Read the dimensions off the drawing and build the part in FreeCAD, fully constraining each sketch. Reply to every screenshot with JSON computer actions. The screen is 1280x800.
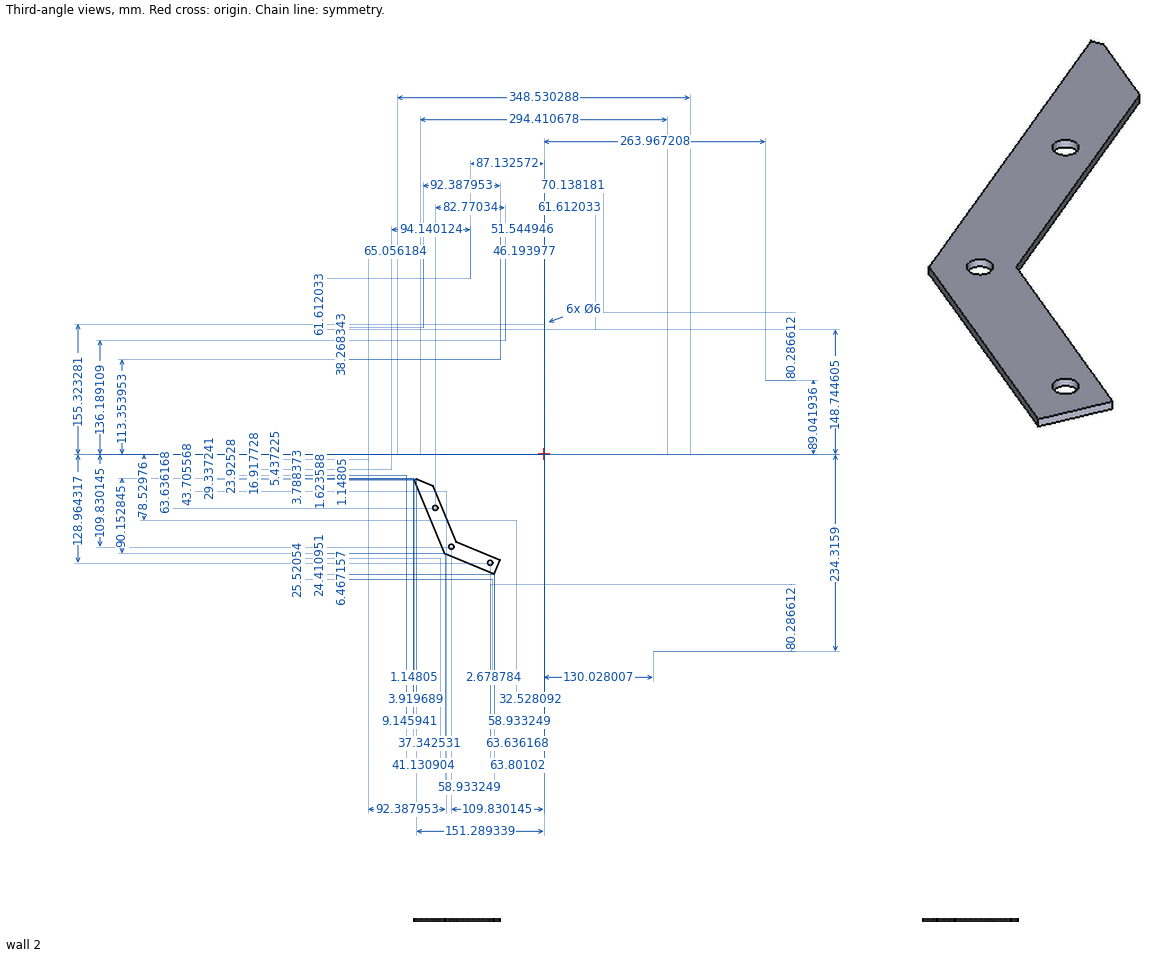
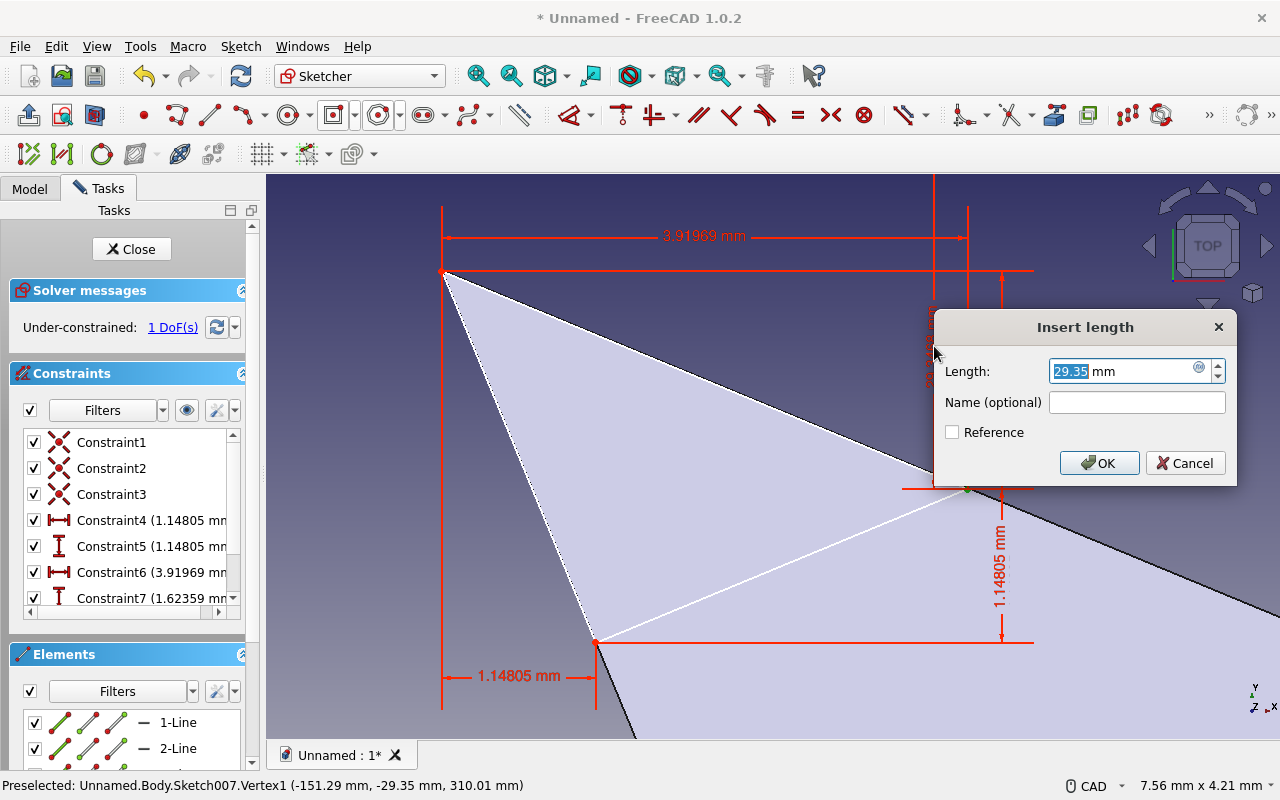
{"action": "type", "text": "29.337241"}
{"action": "key", "text": "Return"}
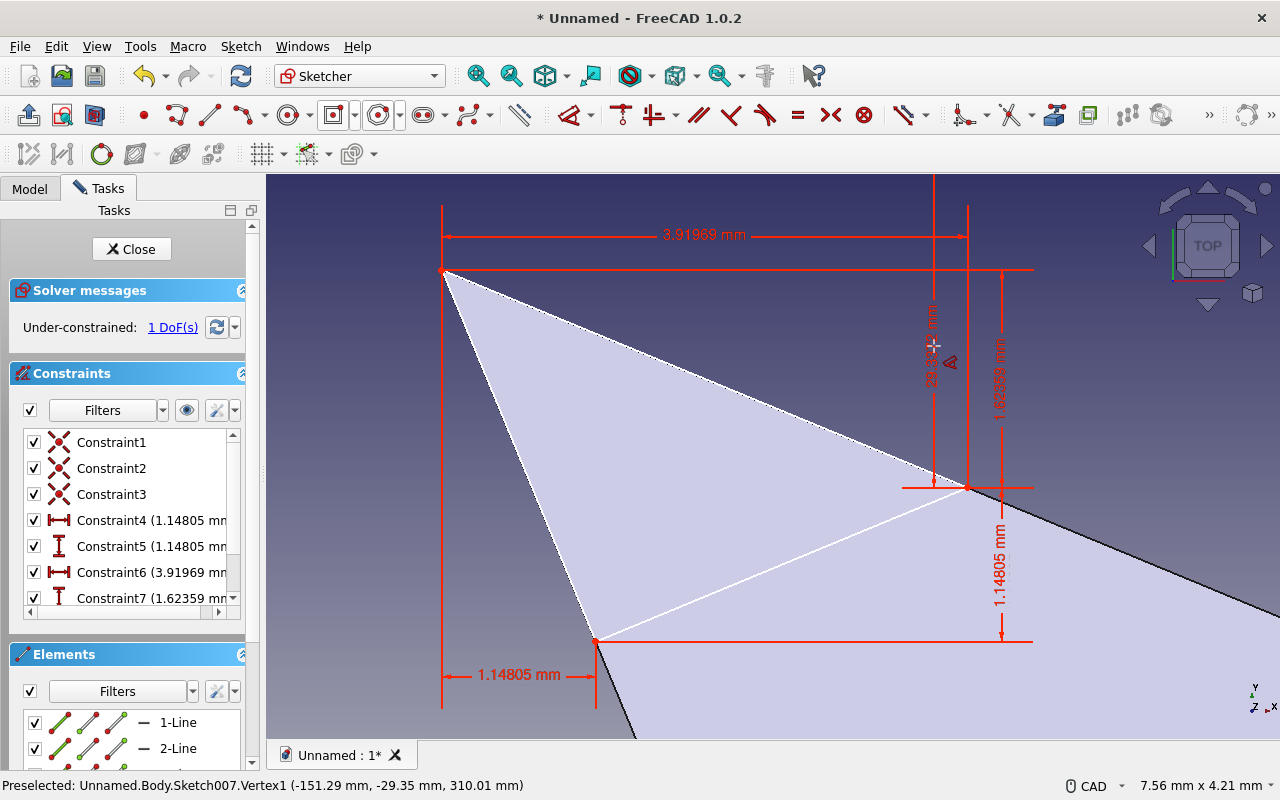
{"action": "left_click", "coordinate": [968, 488]}
{"action": "left_click", "coordinate": [1041, 522]}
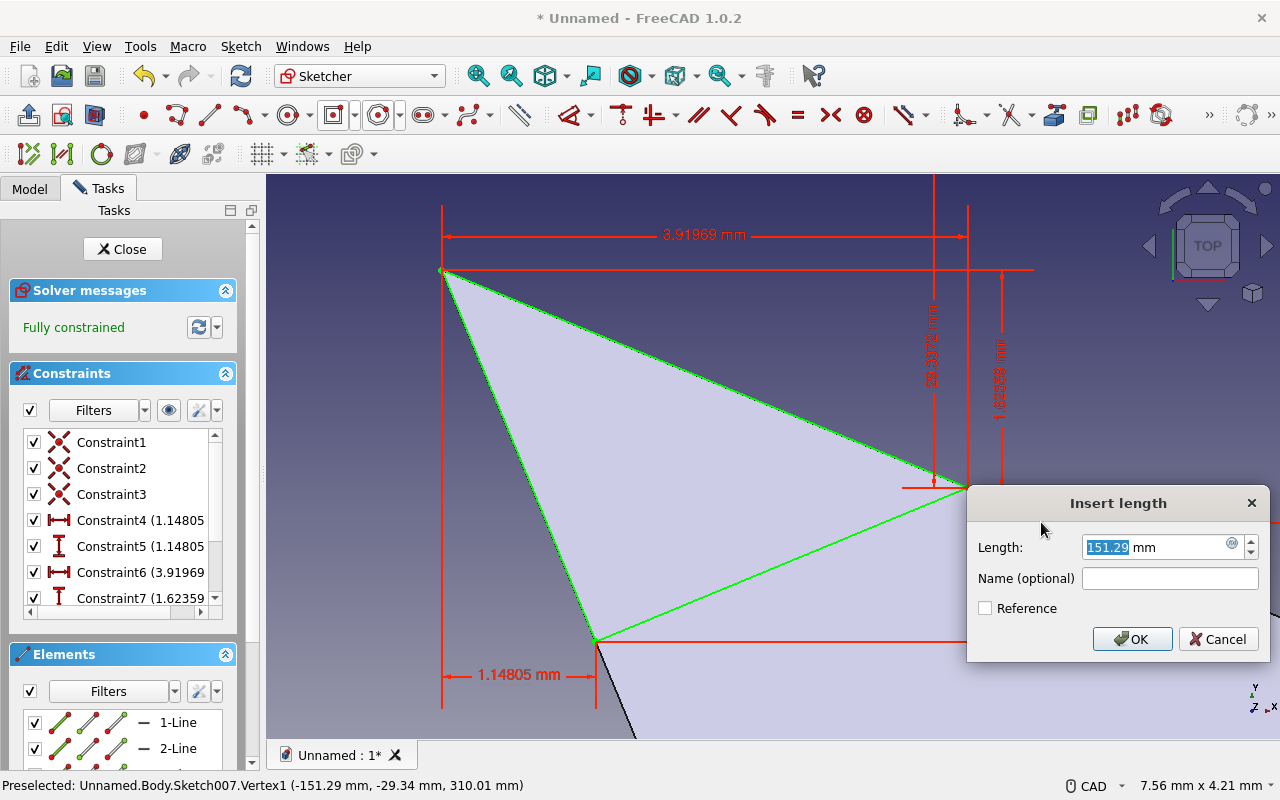
{"action": "type", "text": "151.289339"}
{"action": "key", "text": "Return"}
{"action": "key", "text": "Escape"}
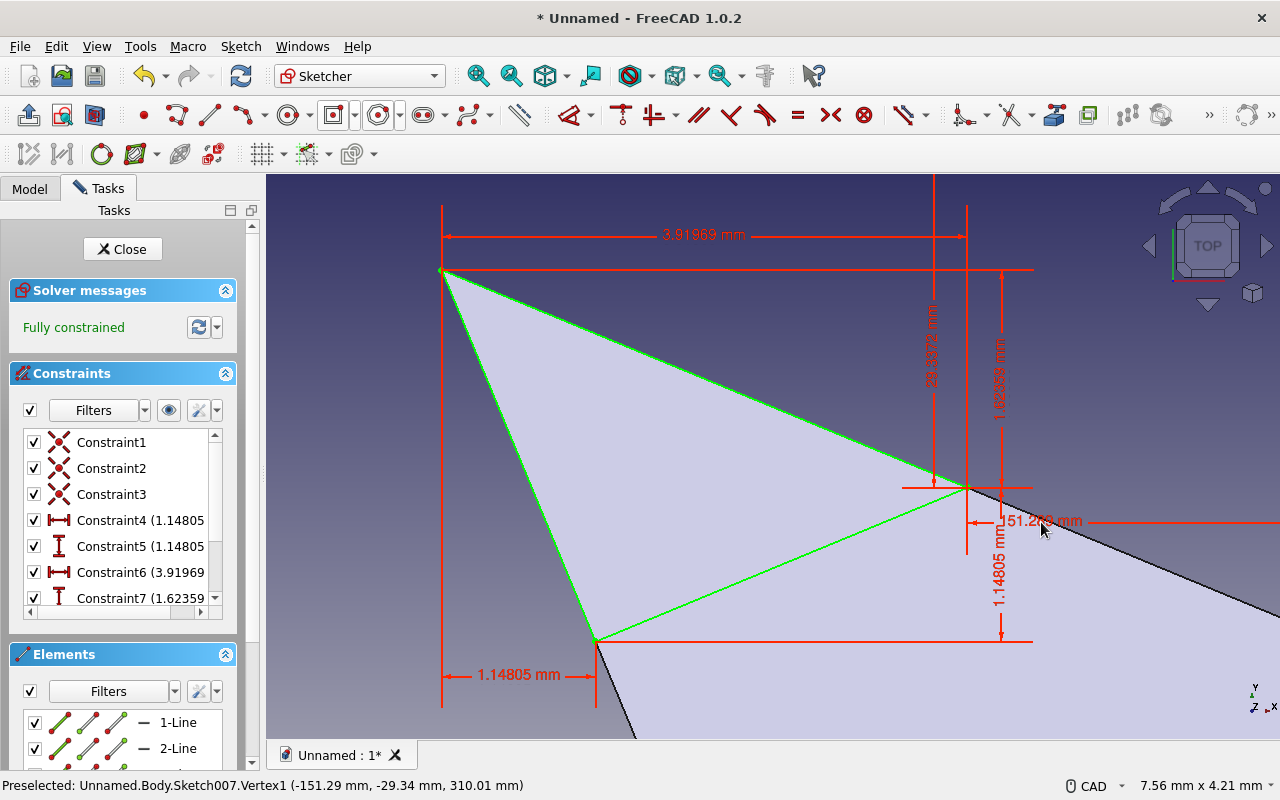
{"action": "left_click", "coordinate": [123, 249]}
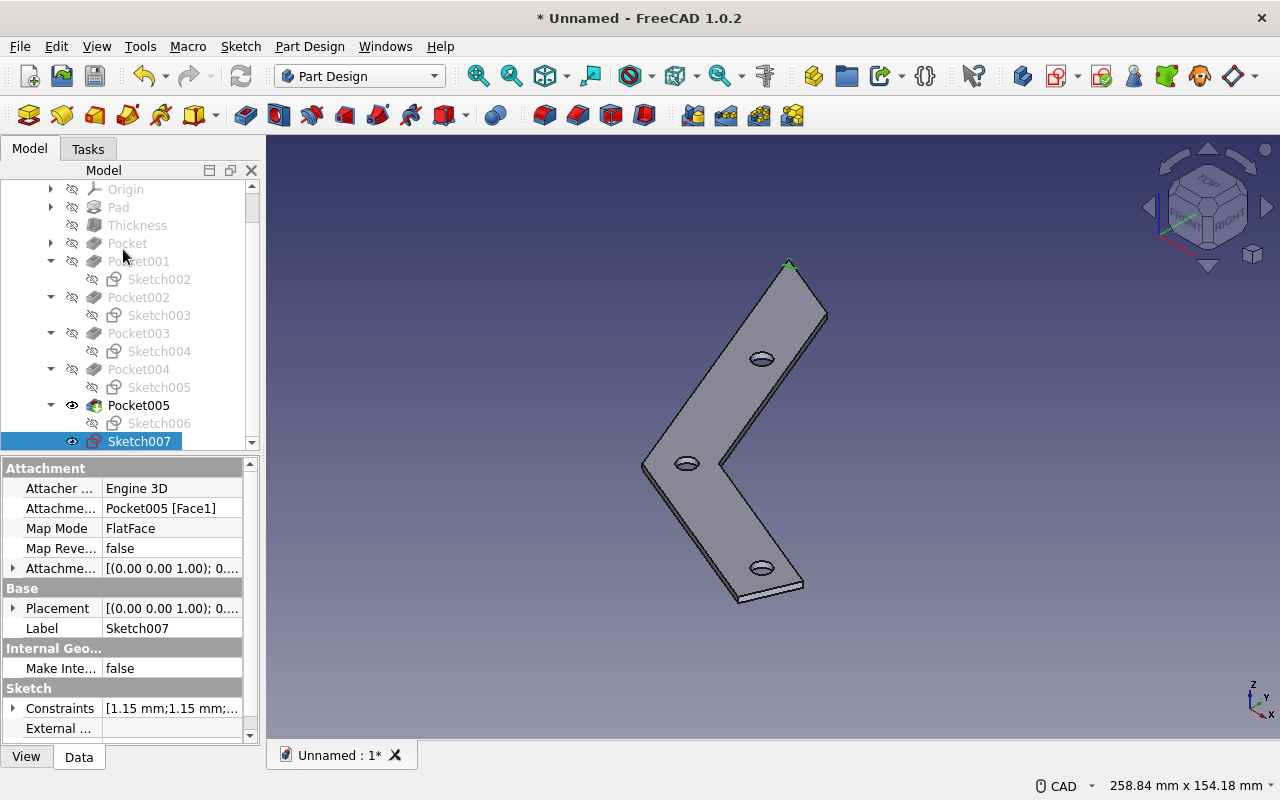
{"action": "left_click", "coordinate": [246, 116]}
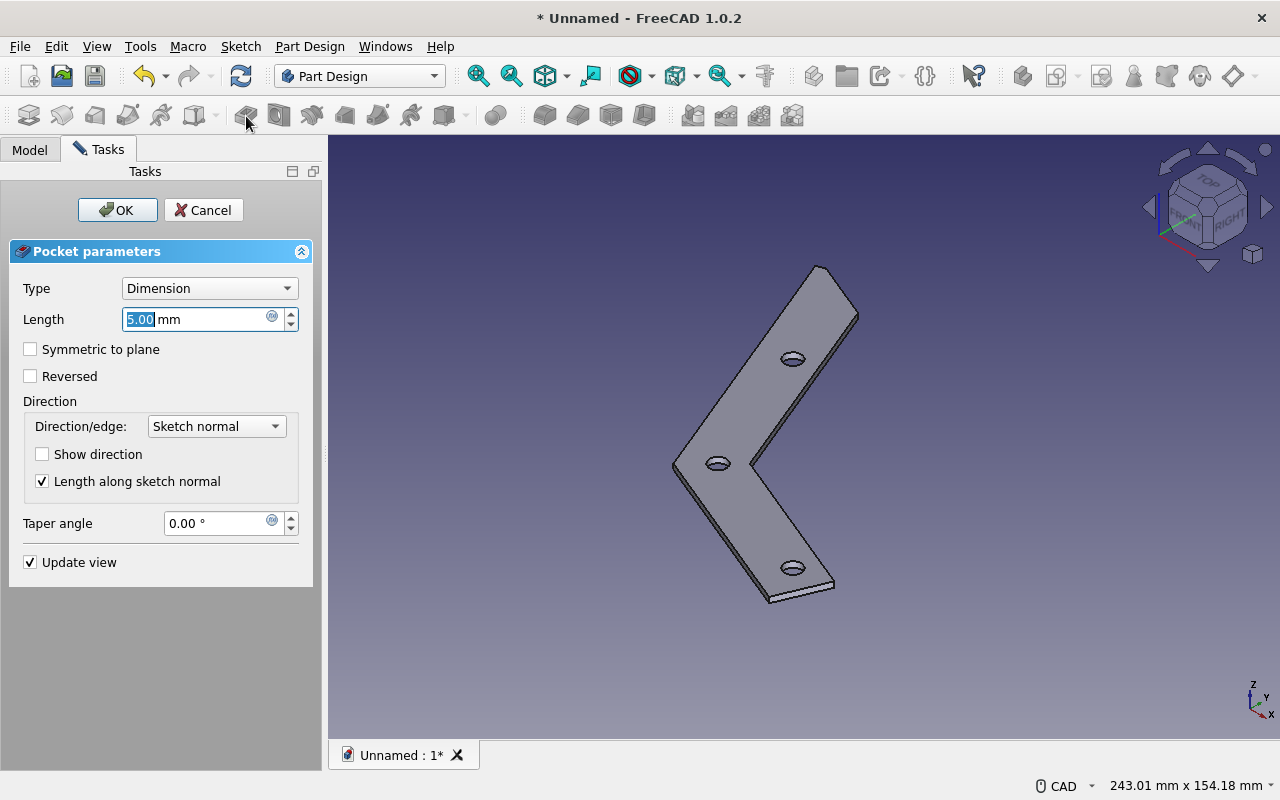
{"action": "left_click", "coordinate": [210, 288]}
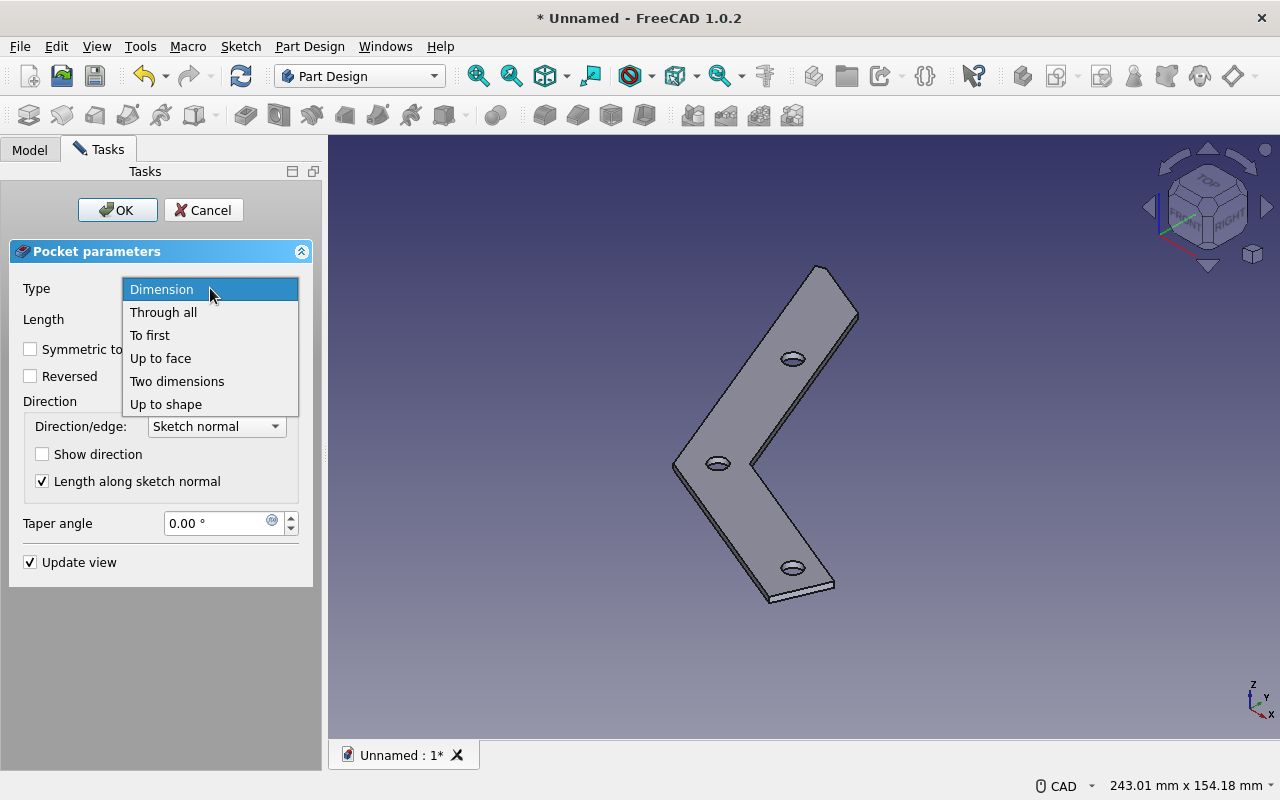
{"action": "left_click", "coordinate": [208, 312]}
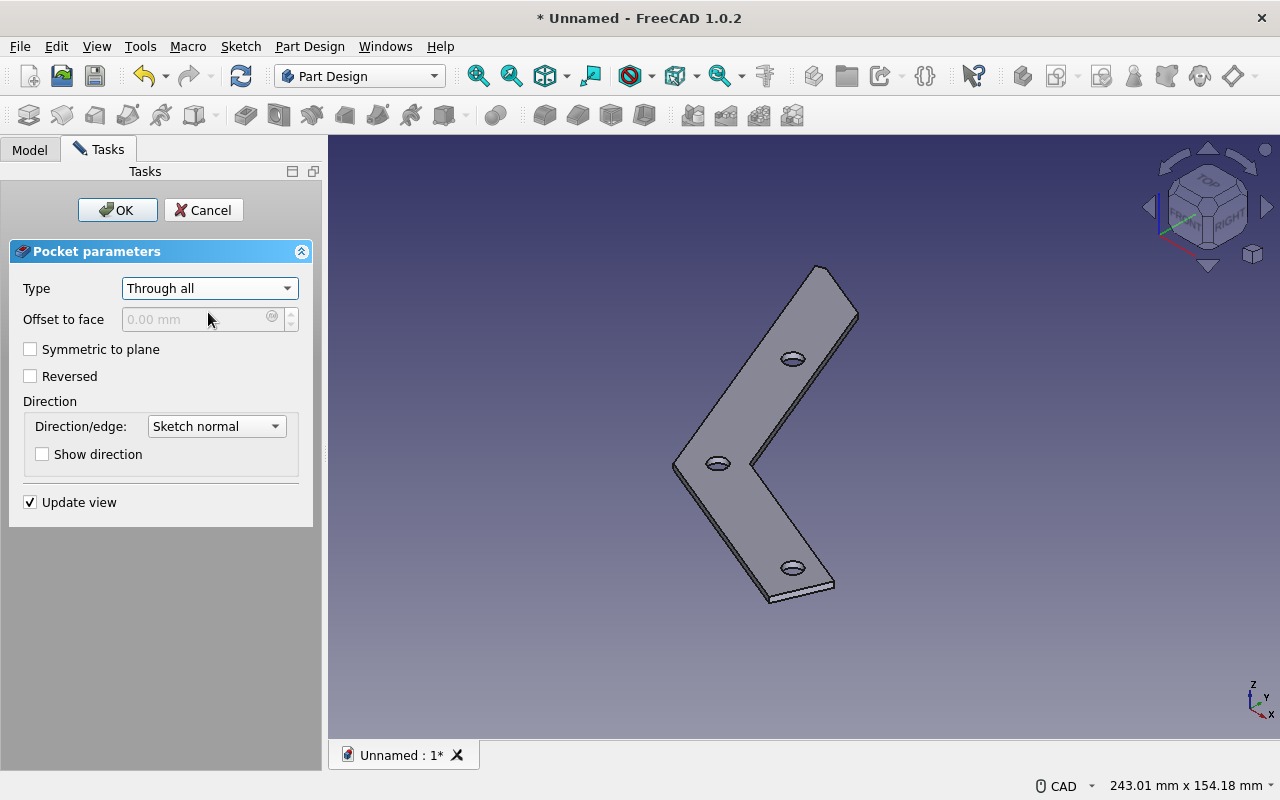
{"action": "left_click", "coordinate": [118, 210]}